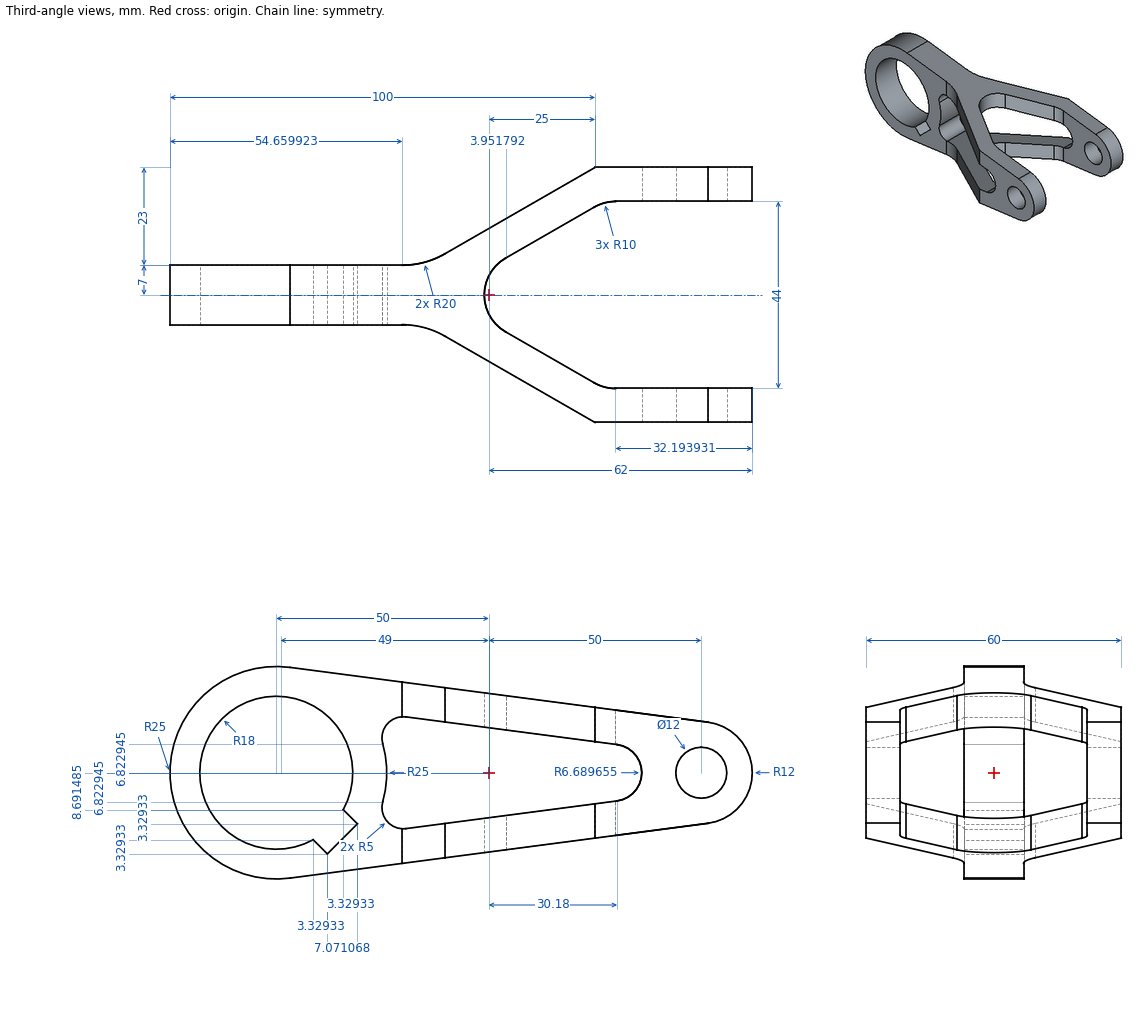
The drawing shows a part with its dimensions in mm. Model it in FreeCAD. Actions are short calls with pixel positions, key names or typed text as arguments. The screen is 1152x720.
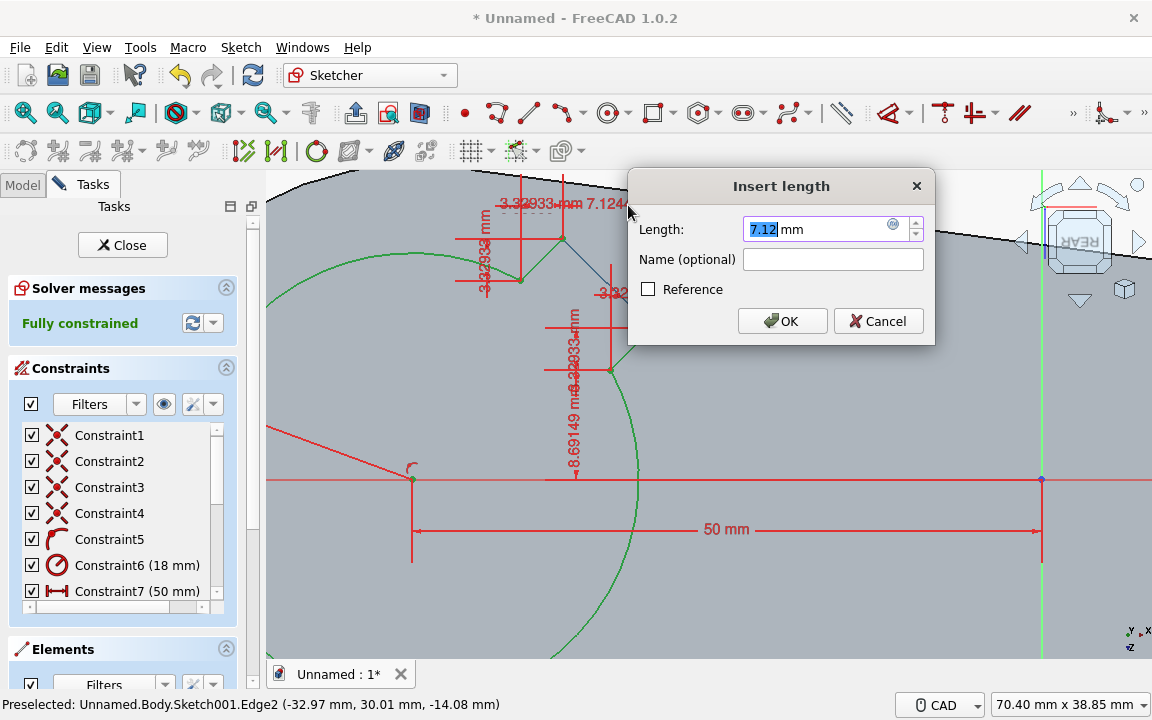
text(7.071068)
key(Return)
key(Escape)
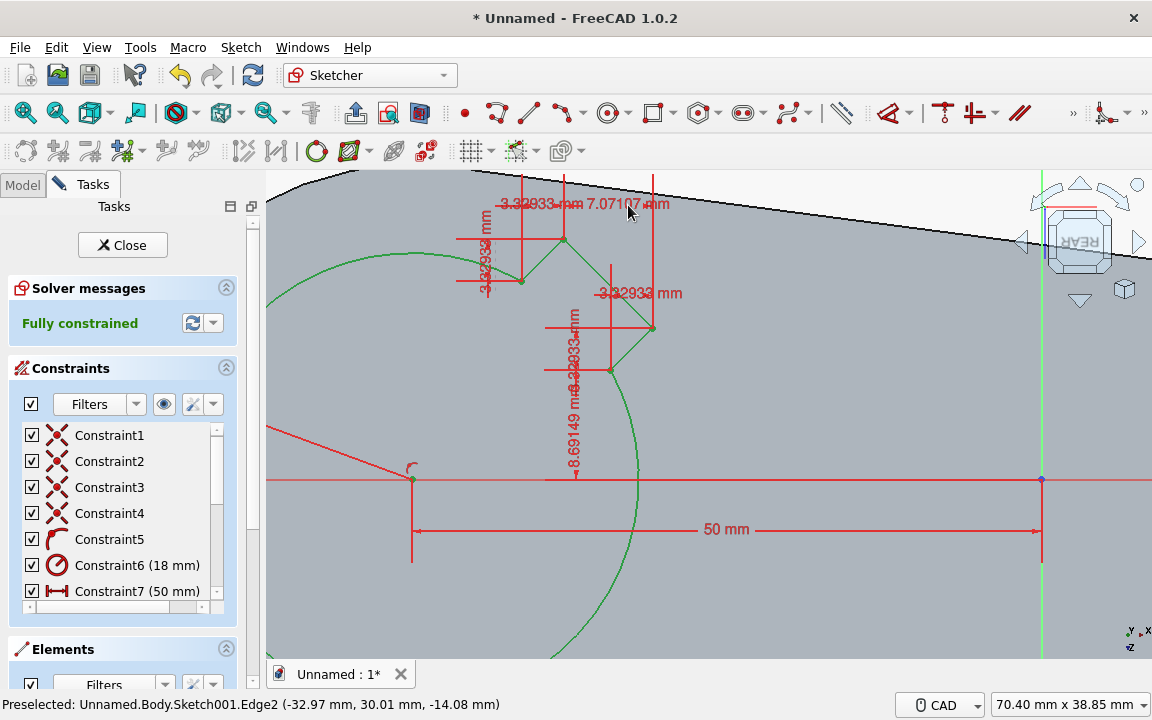
click(123, 245)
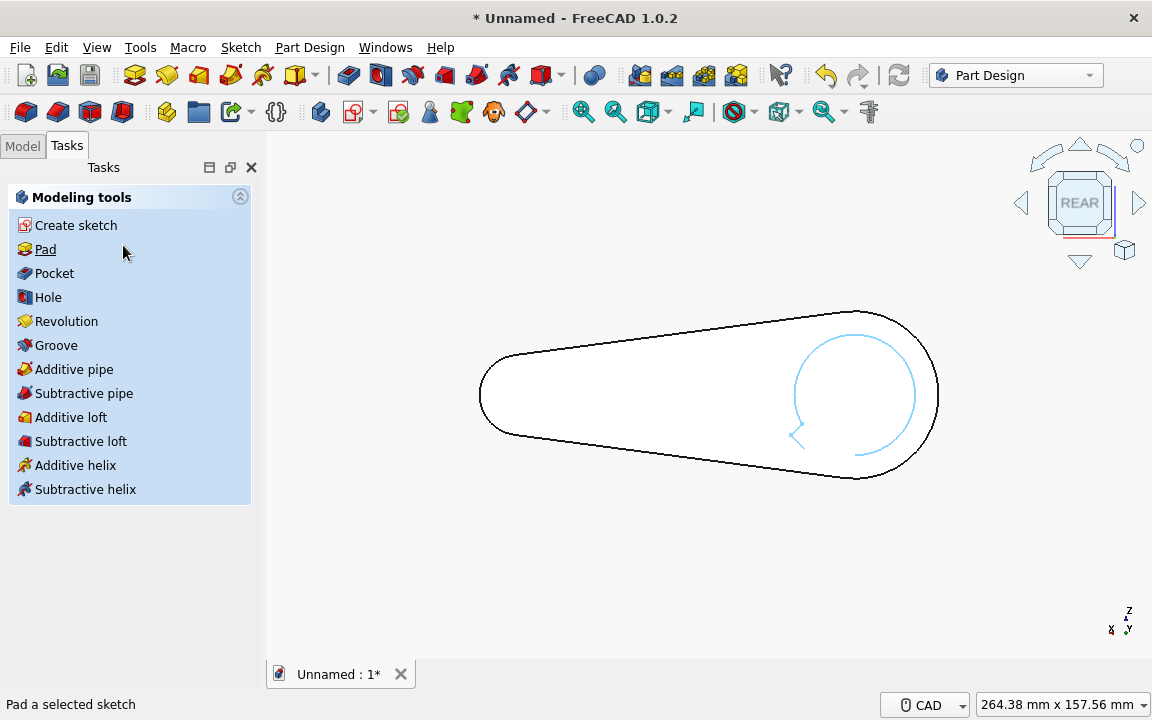
click(350, 76)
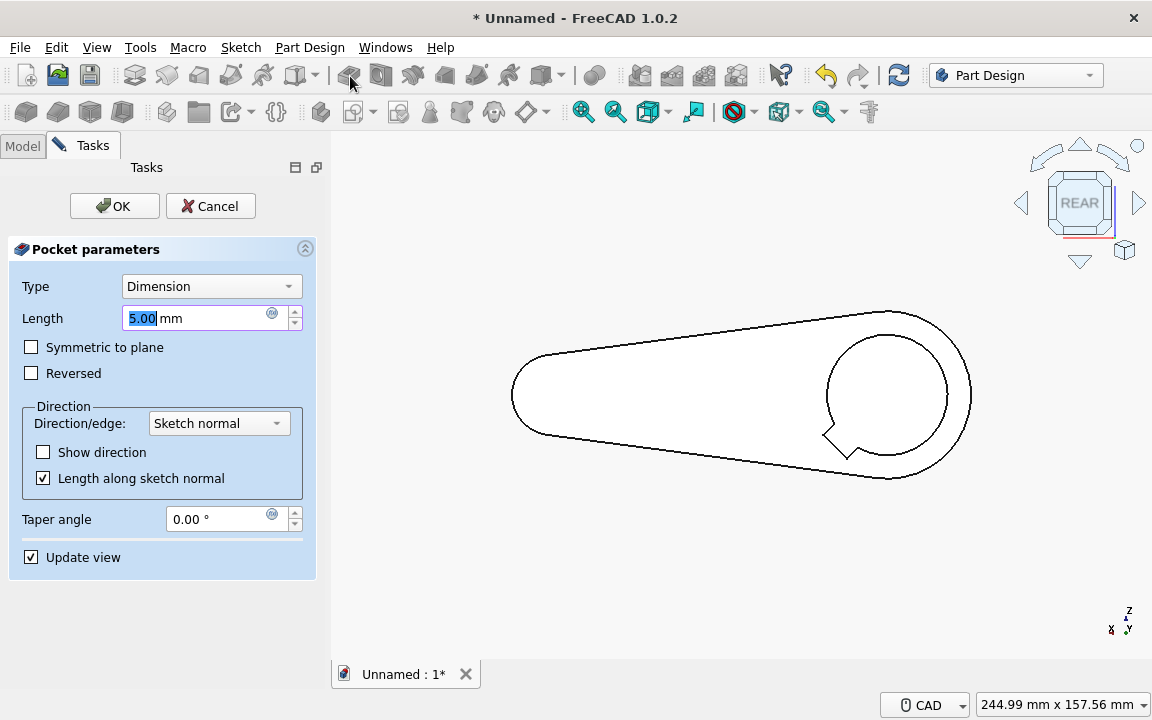
click(212, 286)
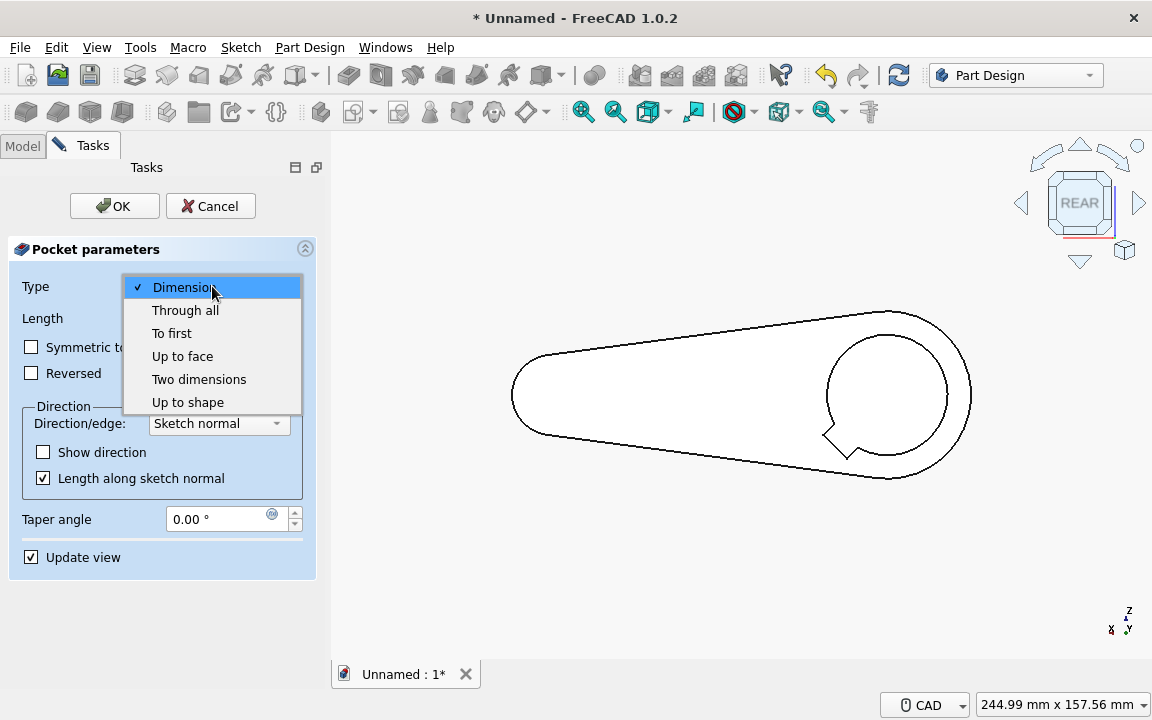
click(212, 310)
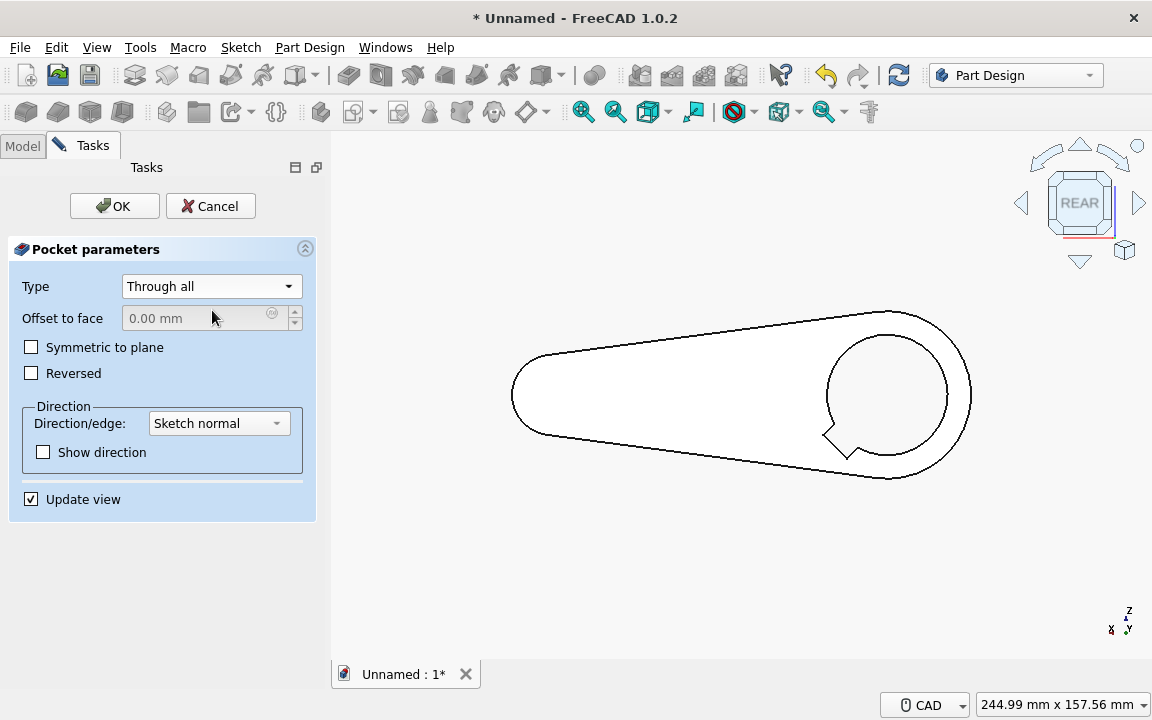
click(115, 206)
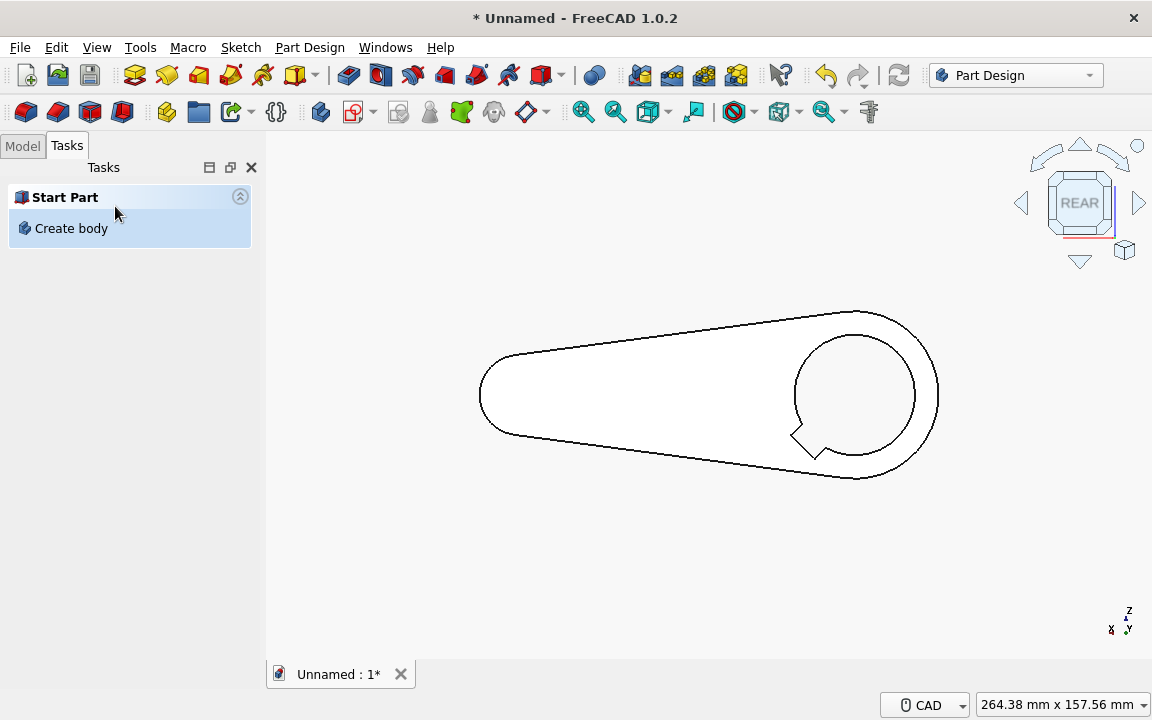
click(709, 394)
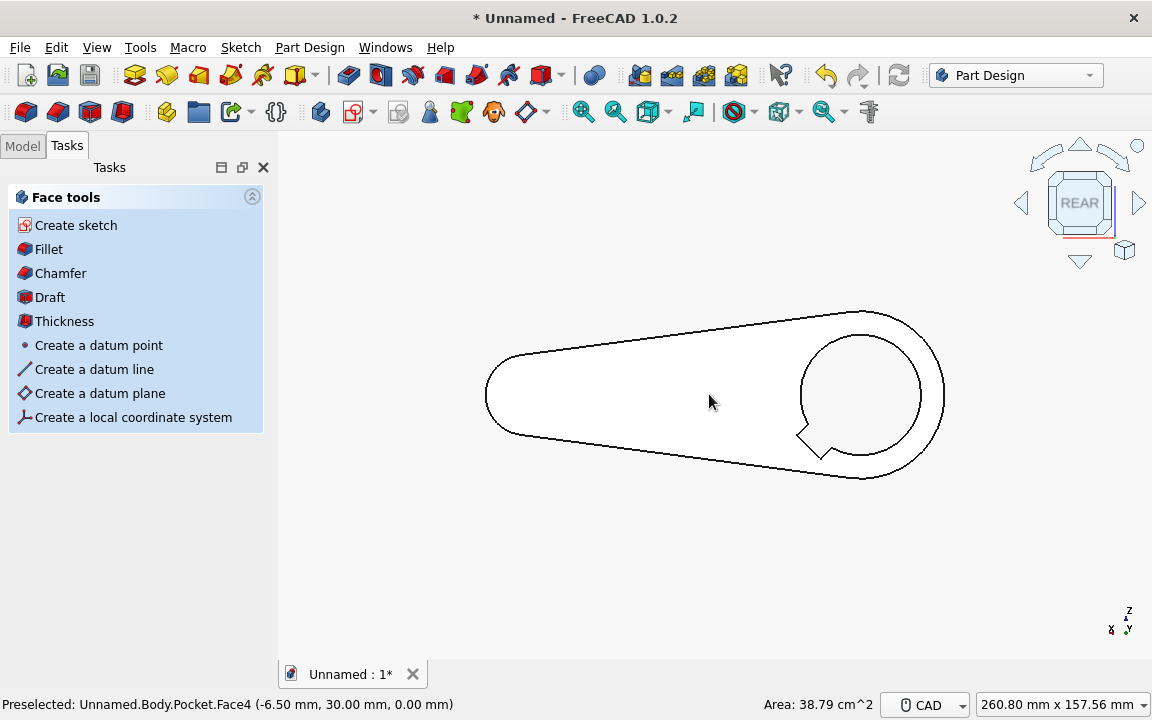
click(354, 112)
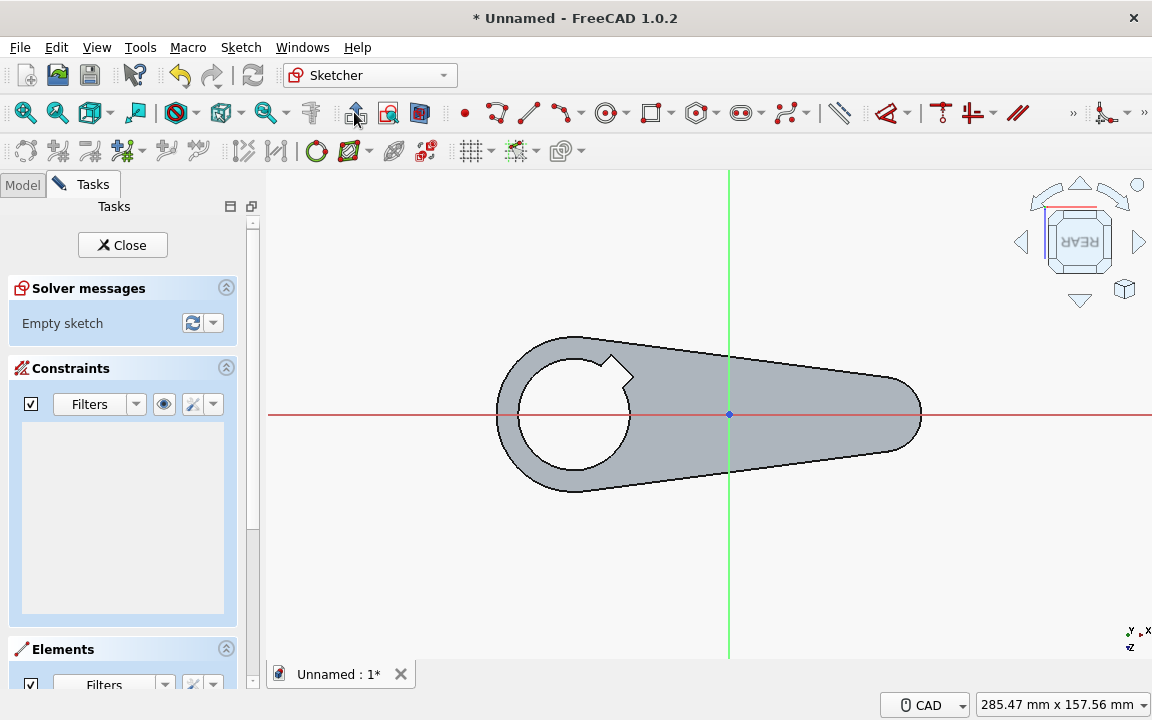
scroll(915, 414, up, 11)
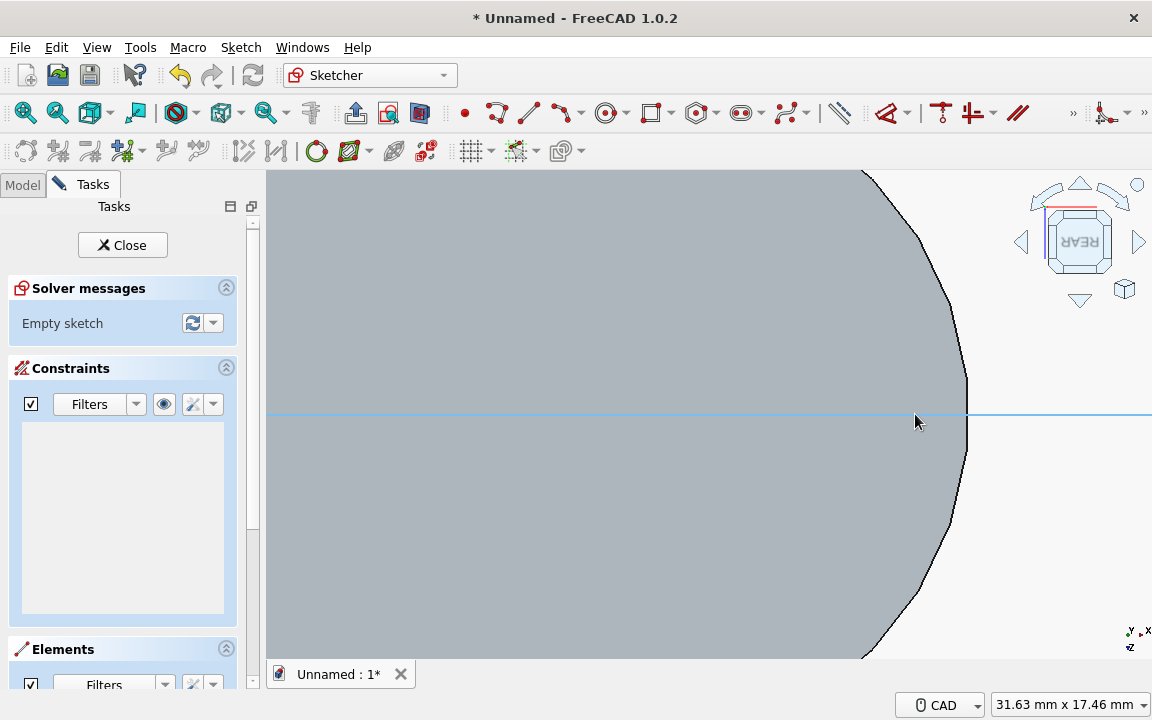
click(606, 114)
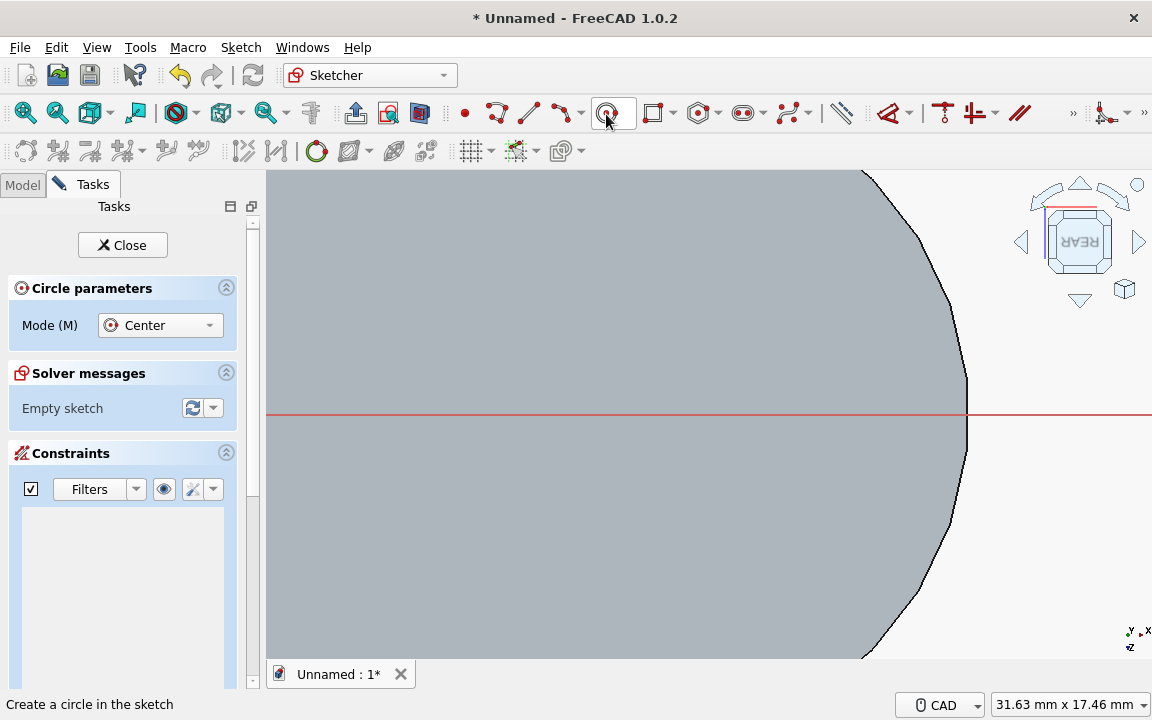
click(632, 414)
move(751, 296)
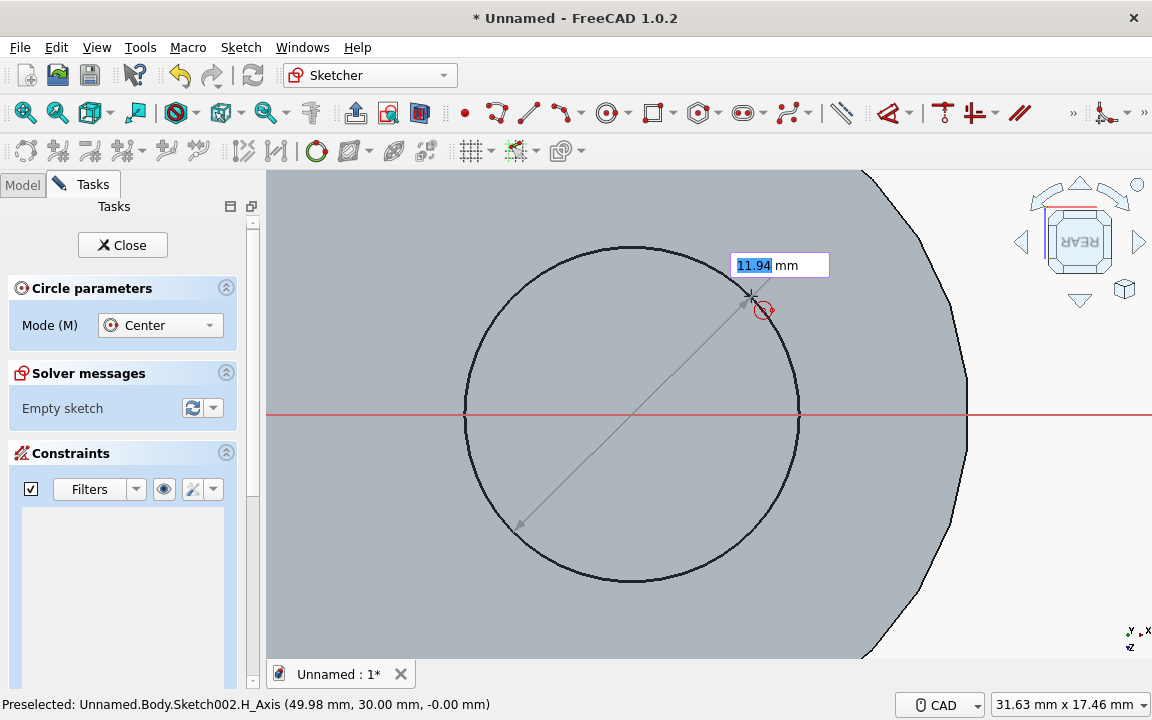
text(12)
key(Return)
key(Escape)